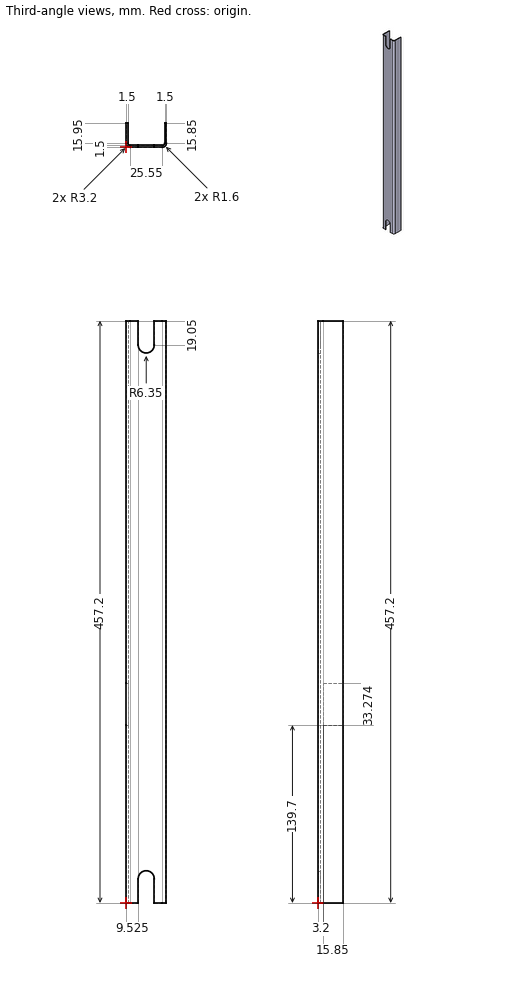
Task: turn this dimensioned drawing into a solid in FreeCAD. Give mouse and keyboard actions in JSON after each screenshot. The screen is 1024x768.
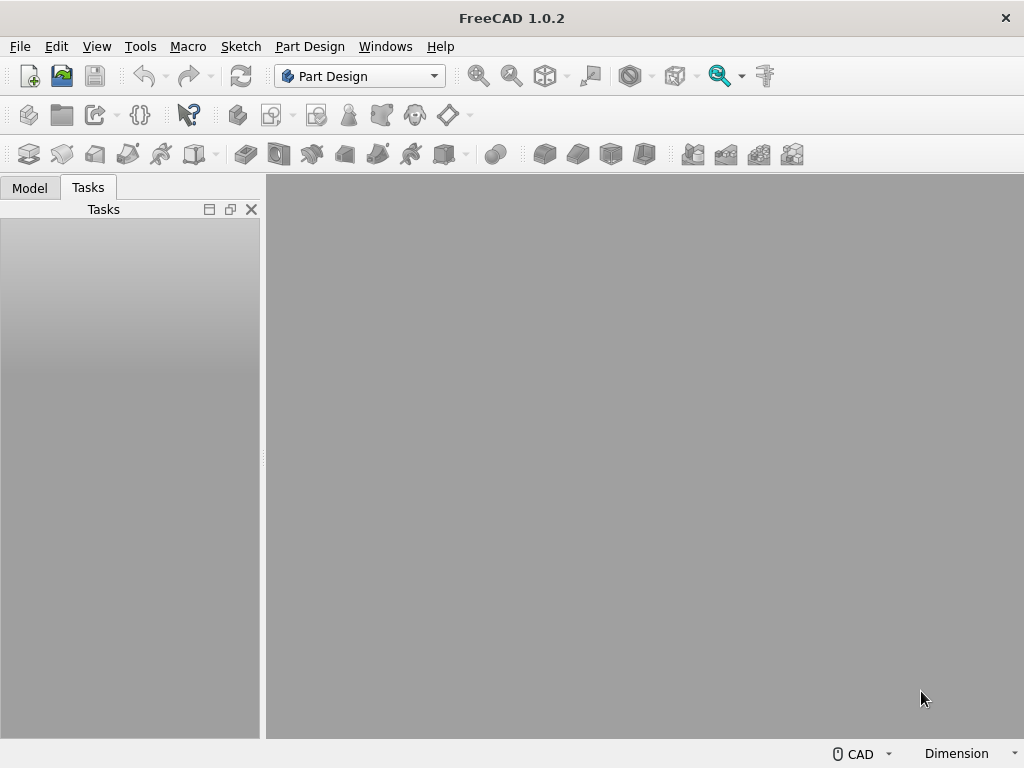
{"action": "key", "text": "ctrl+n"}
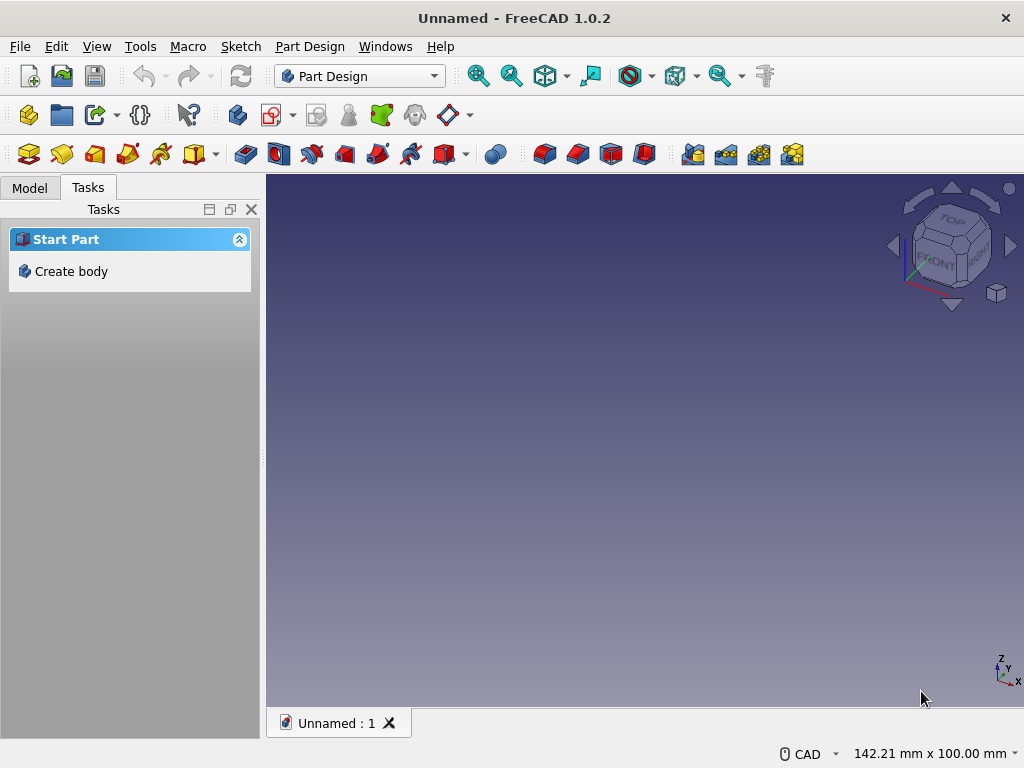
{"action": "left_click", "coordinate": [270, 116]}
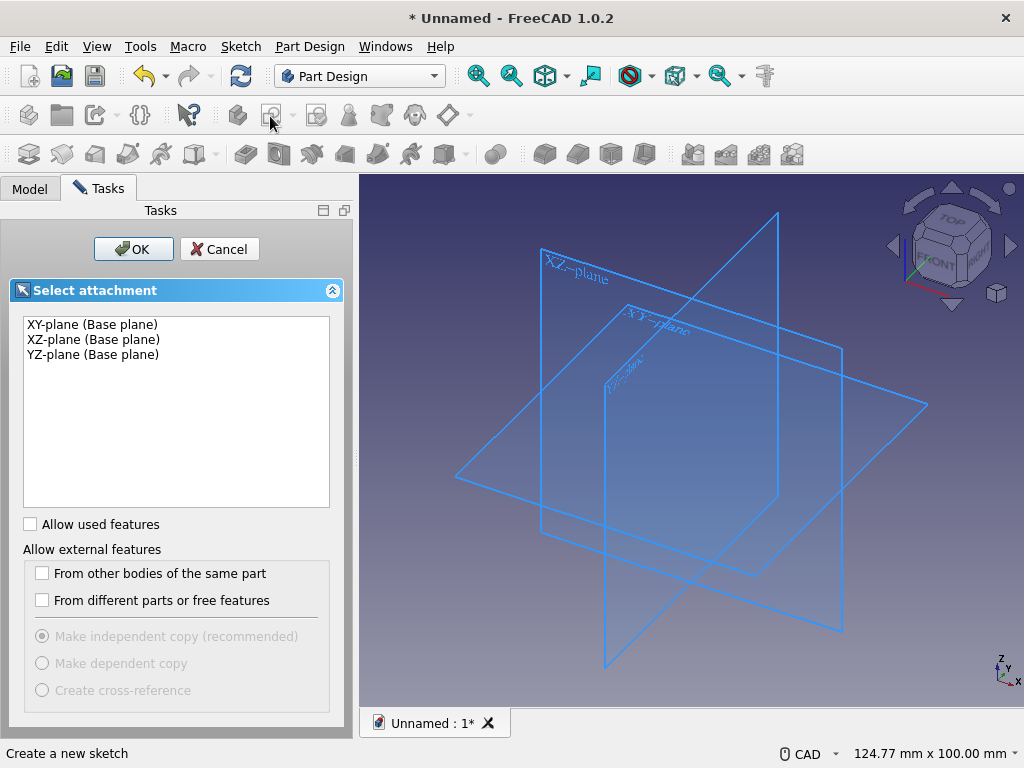
{"action": "left_click", "coordinate": [84, 324]}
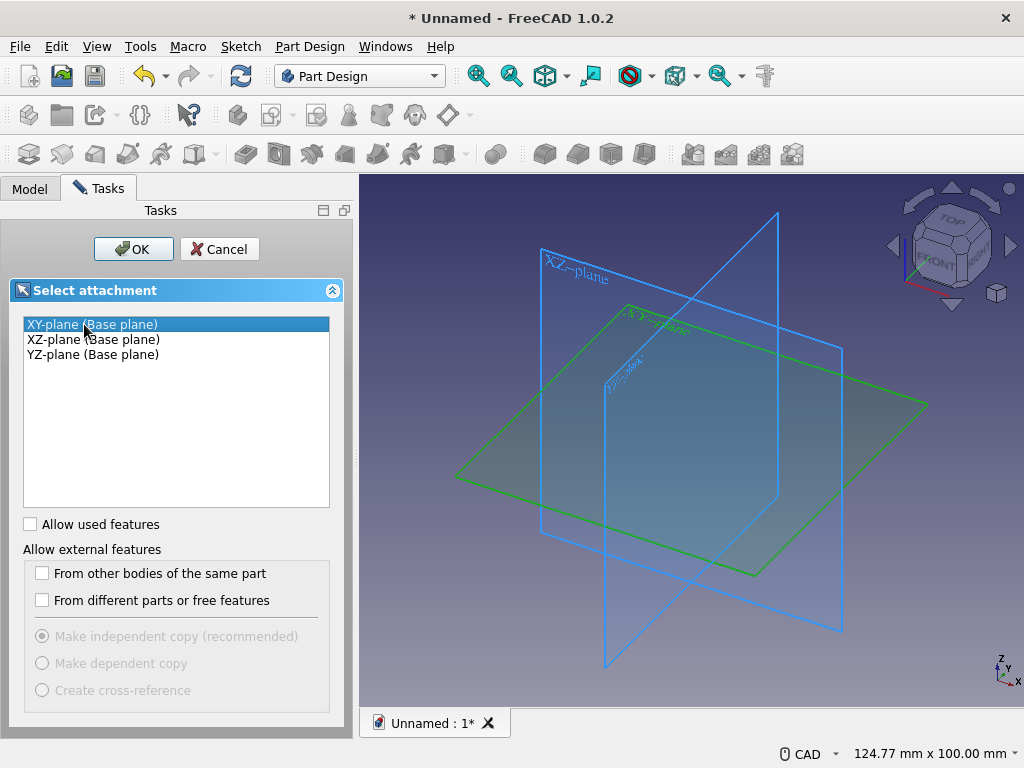
{"action": "left_click", "coordinate": [134, 249]}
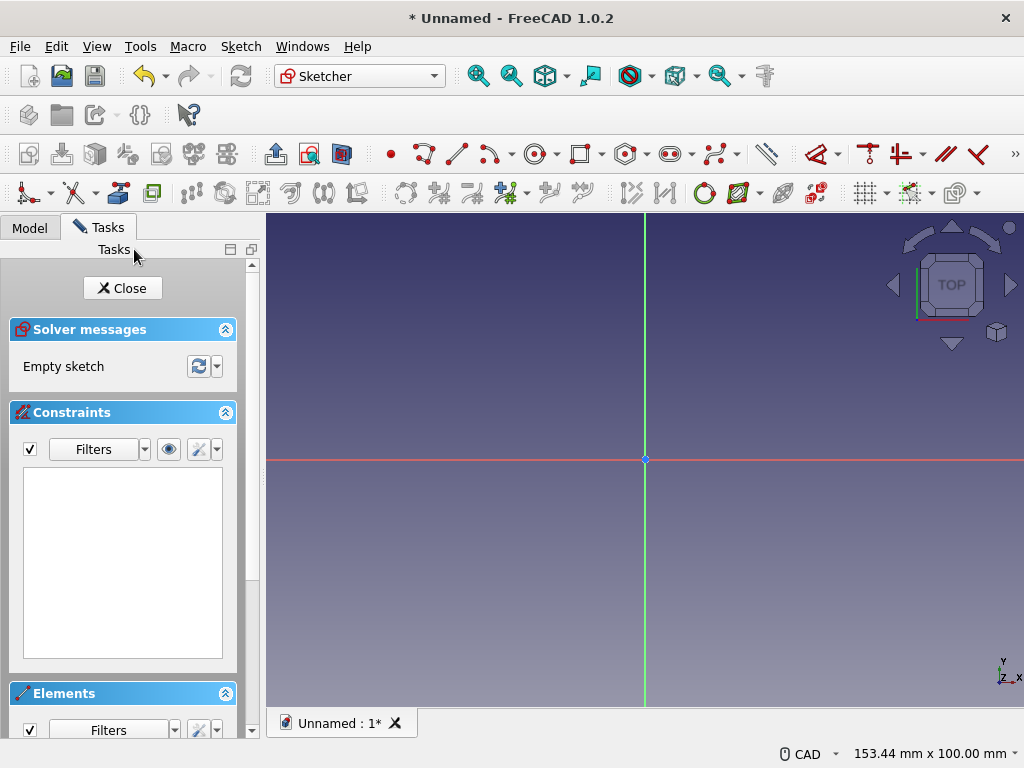
{"action": "scroll", "coordinate": [809, 386], "scroll_direction": "up", "scroll_amount": 5}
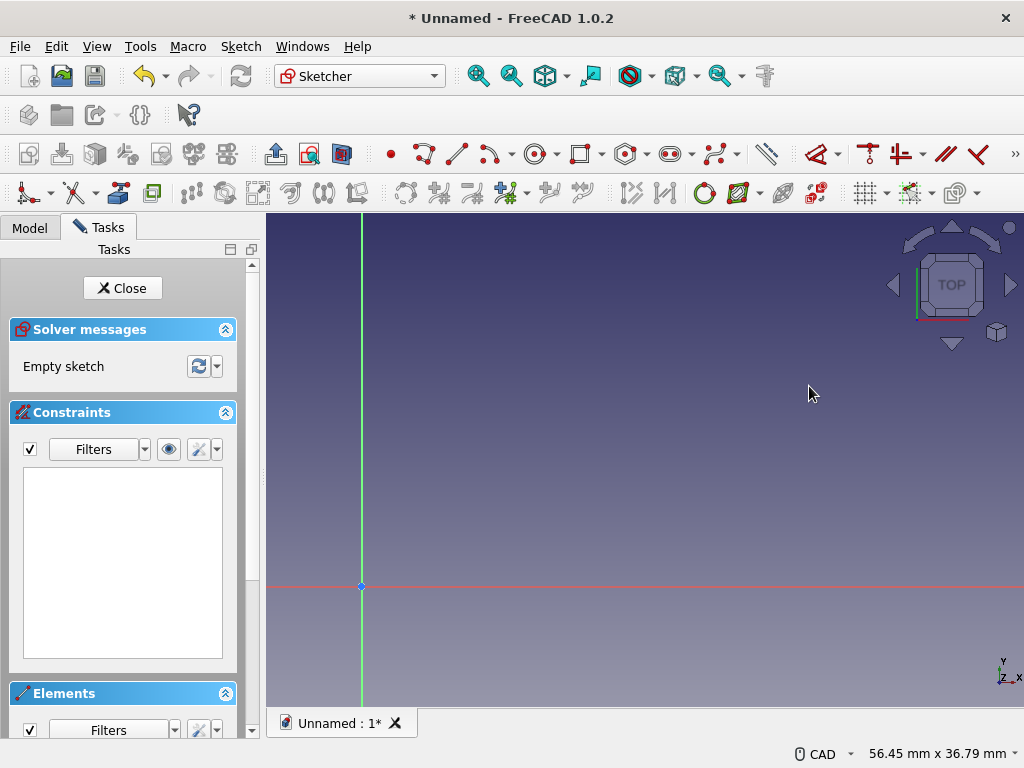
{"action": "key", "text": "g l"}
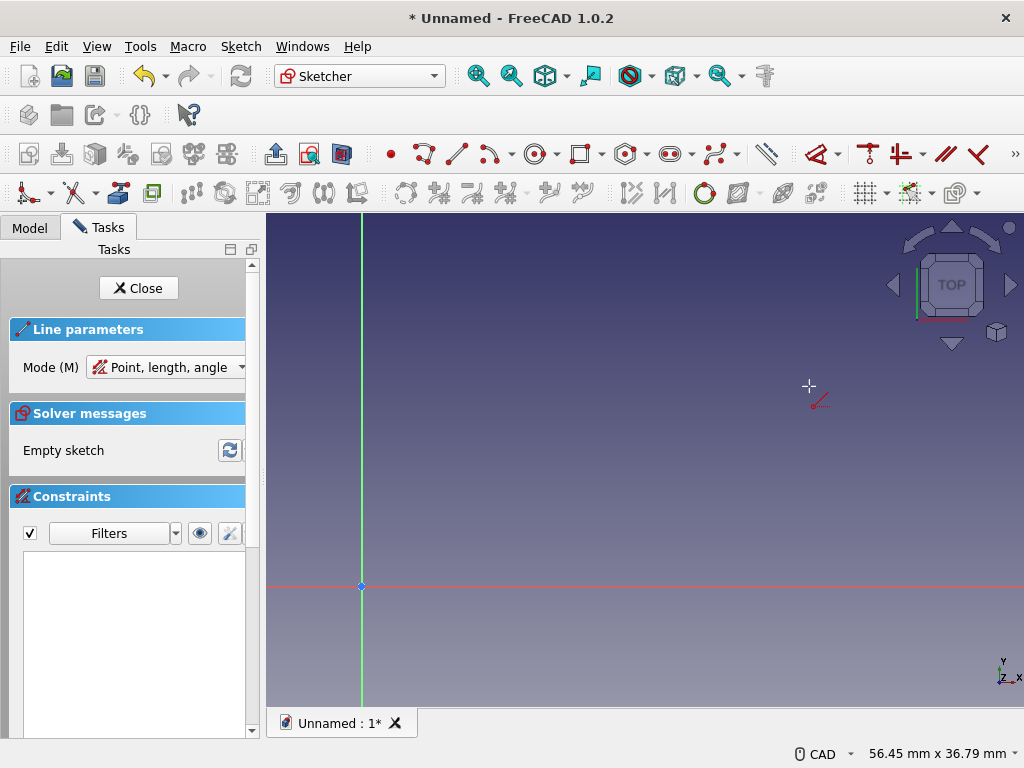
{"action": "left_click", "coordinate": [747, 566]}
{"action": "left_click", "coordinate": [404, 566]}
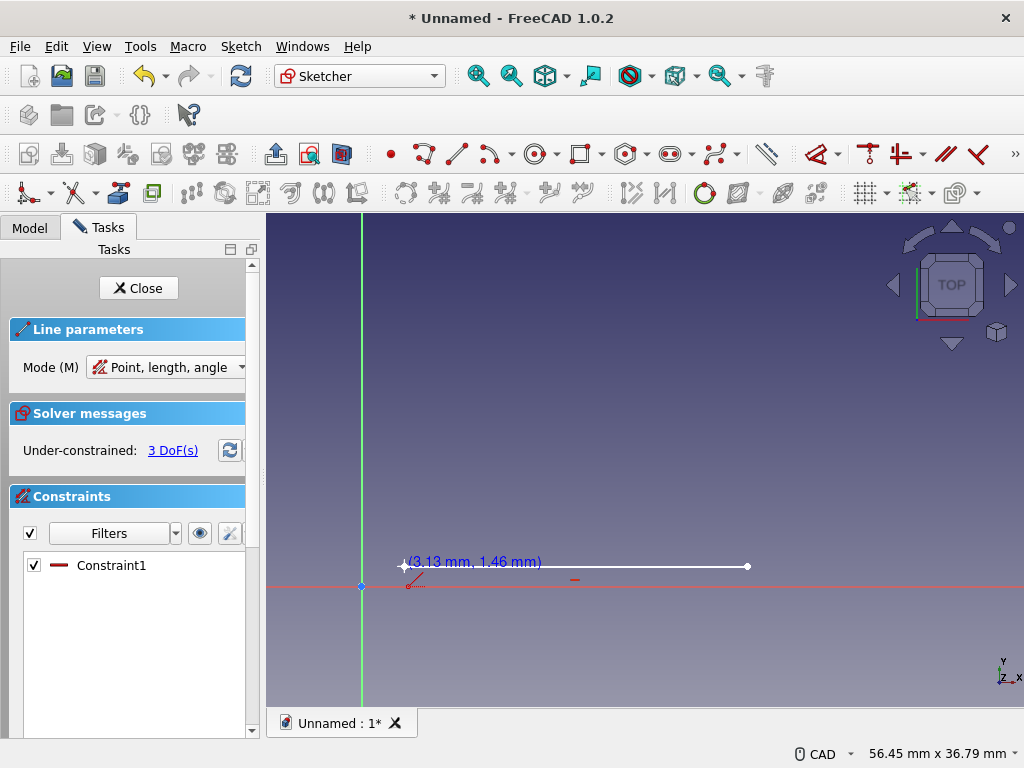
{"action": "key", "text": "g m"}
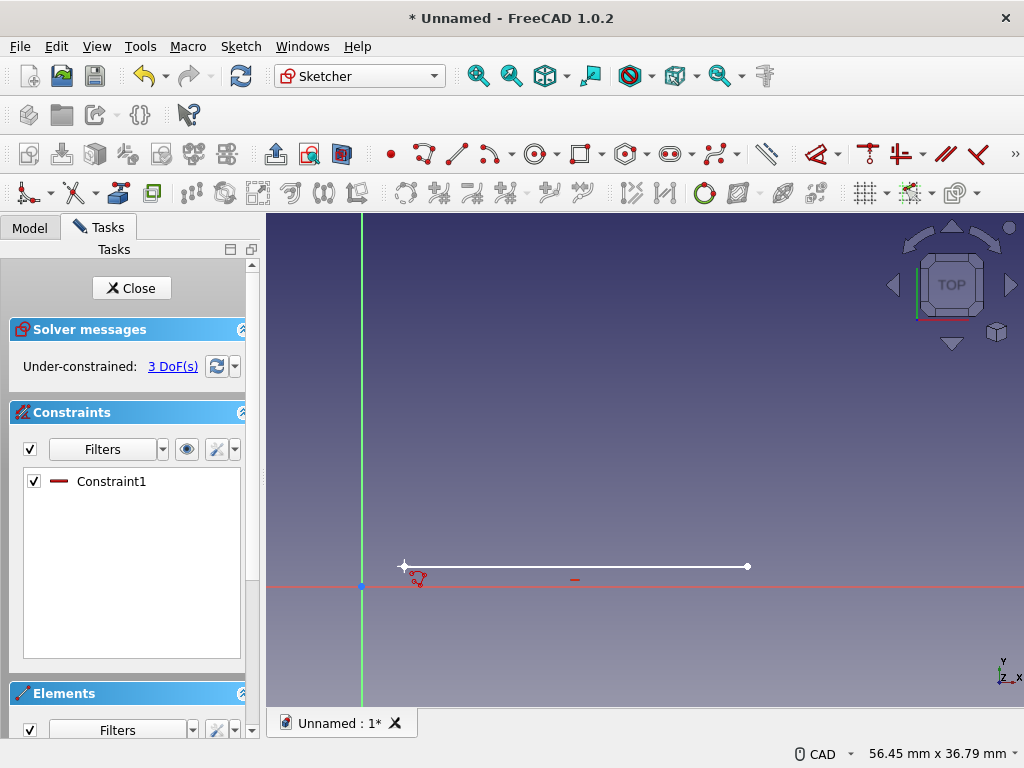
{"action": "left_click", "coordinate": [382, 545]}
{"action": "left_click", "coordinate": [382, 331]}
{"action": "left_click", "coordinate": [362, 331]}
{"action": "left_click", "coordinate": [371, 544]}
{"action": "right_click", "coordinate": [371, 544]}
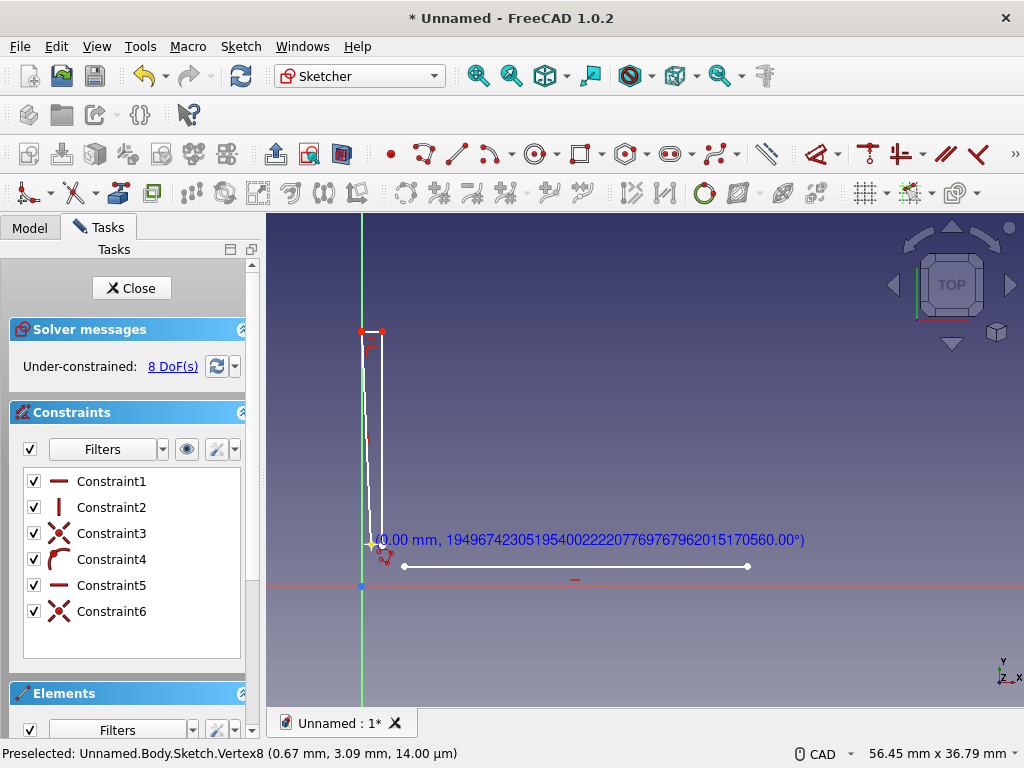
{"action": "key", "text": "g l"}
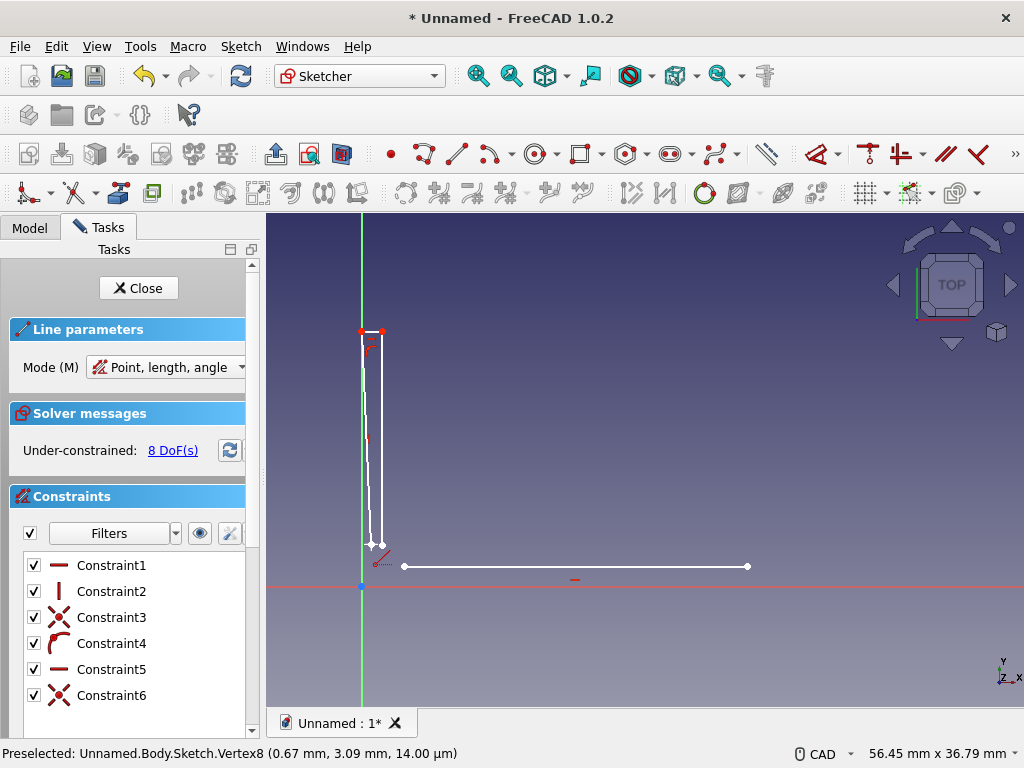
{"action": "left_click", "coordinate": [405, 587]}
{"action": "left_click", "coordinate": [745, 578]}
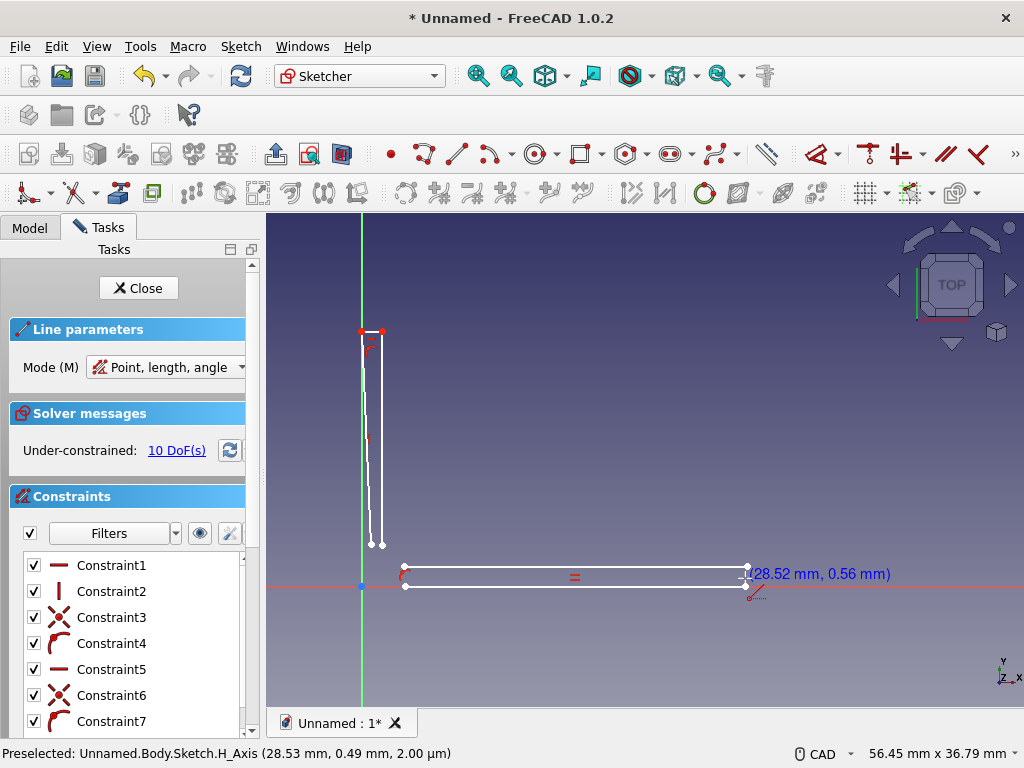
{"action": "key", "text": "g m"}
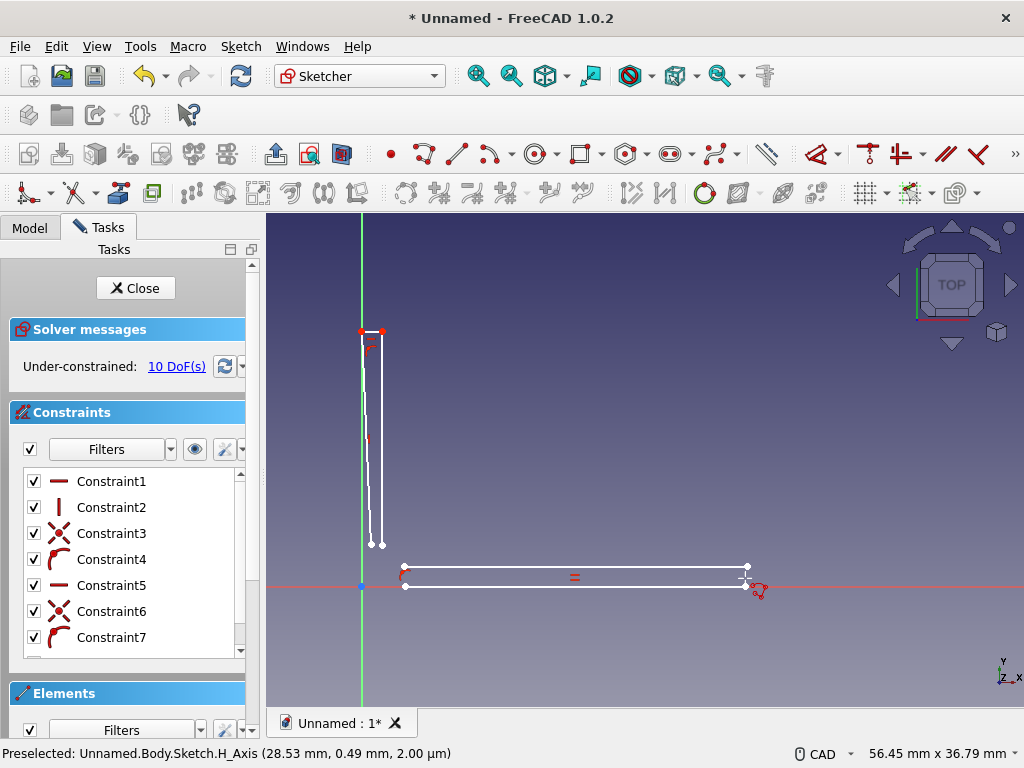
{"action": "left_click", "coordinate": [788, 544]}
{"action": "left_click", "coordinate": [788, 331]}
{"action": "left_click", "coordinate": [768, 331]}
{"action": "left_click", "coordinate": [768, 545]}
{"action": "right_click", "coordinate": [768, 545]}